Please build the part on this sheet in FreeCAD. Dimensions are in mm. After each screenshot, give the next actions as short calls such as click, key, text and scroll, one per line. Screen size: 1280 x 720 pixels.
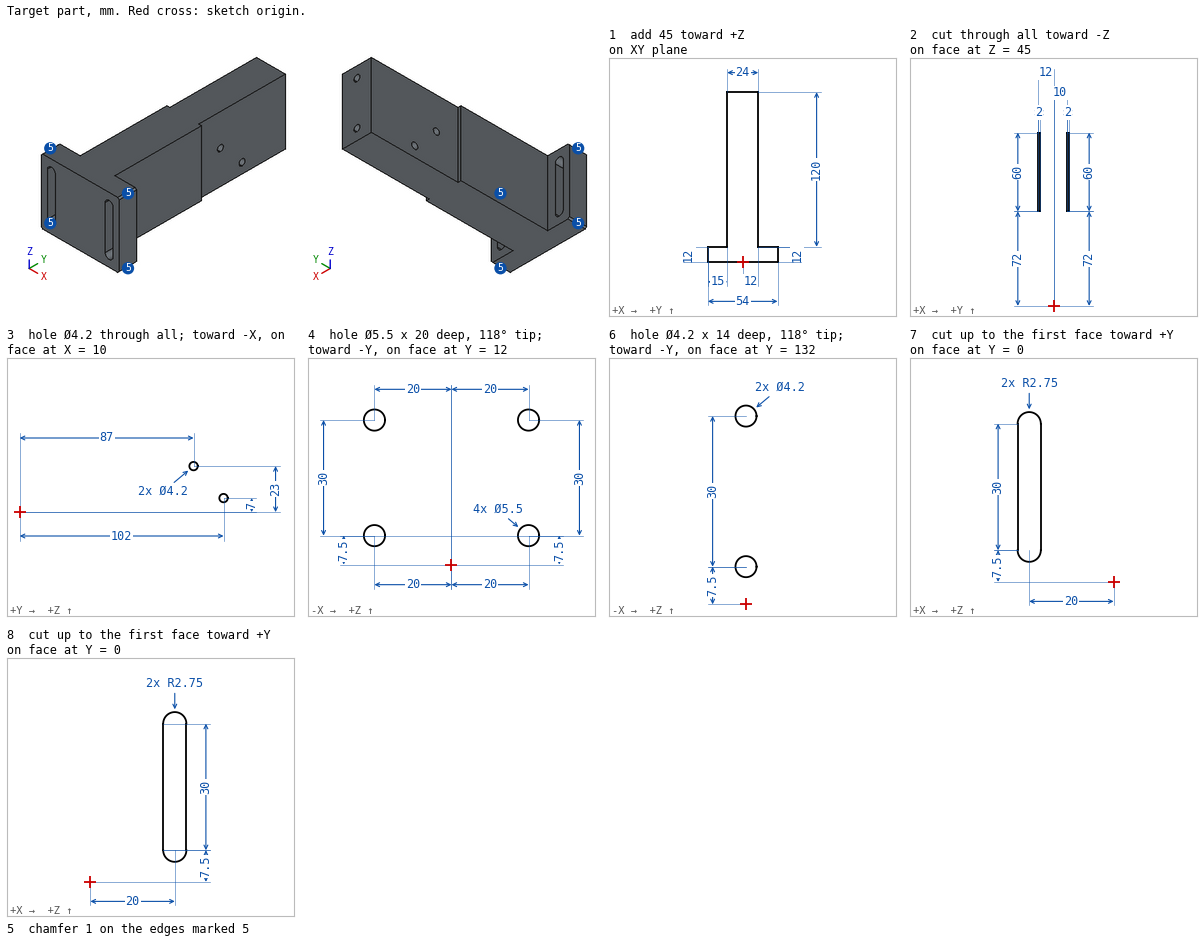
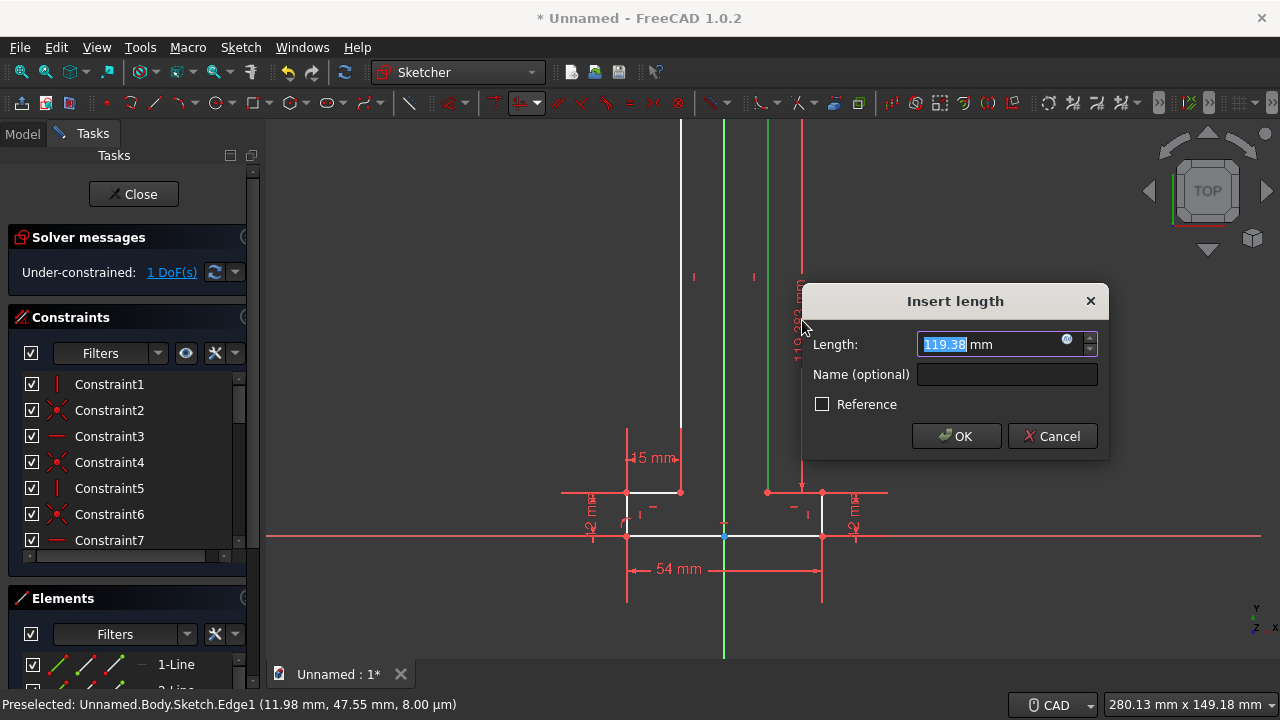
text(120)
key(Return)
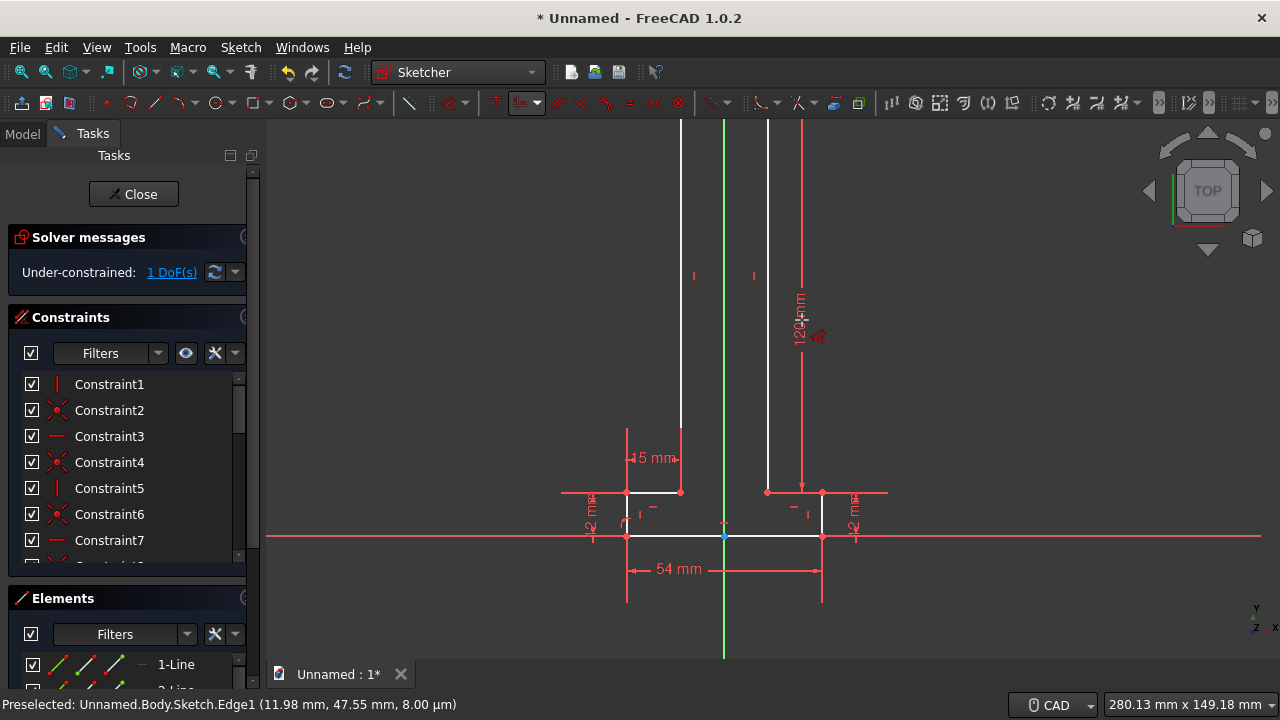
click(768, 493)
click(756, 570)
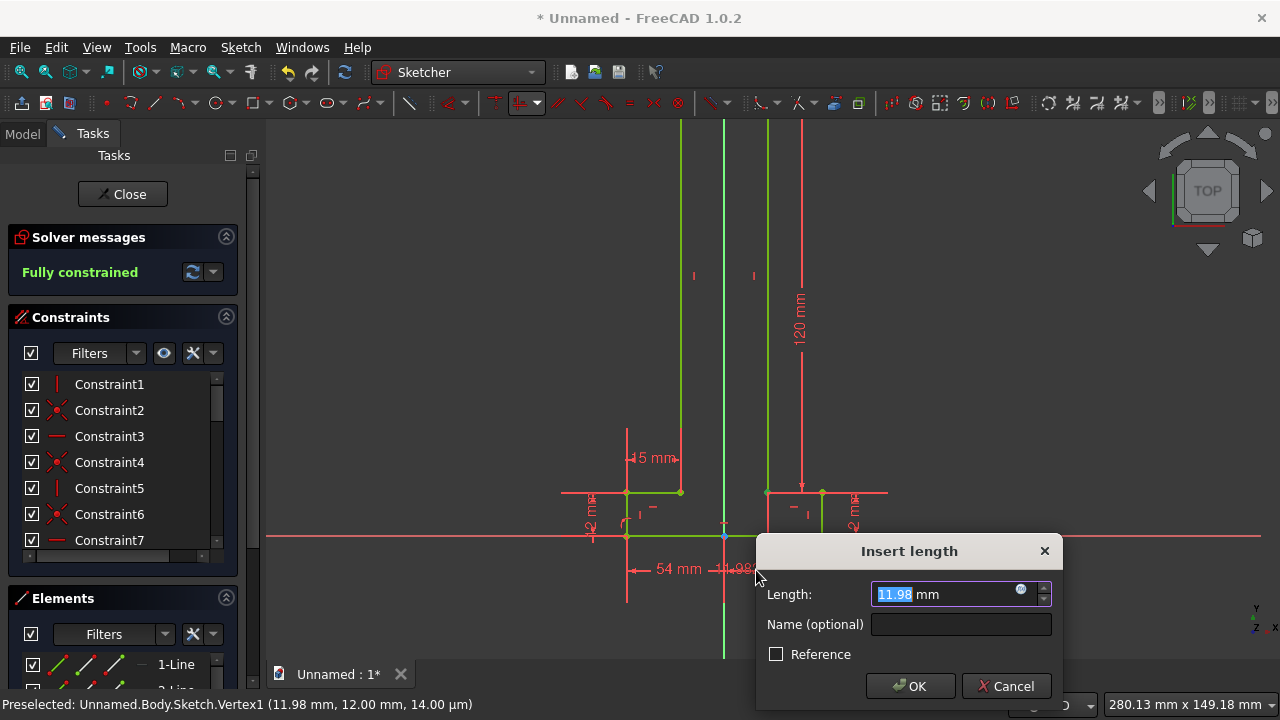
text(12)
key(Return)
key(Escape)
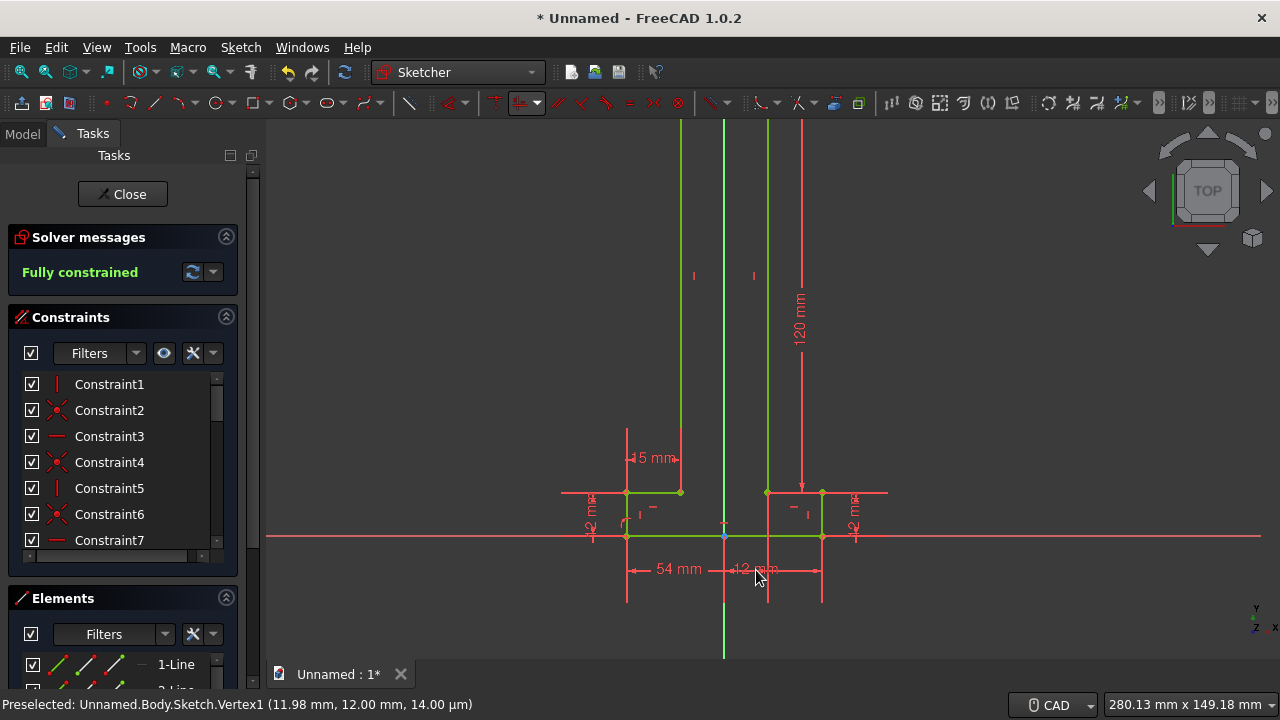
click(123, 194)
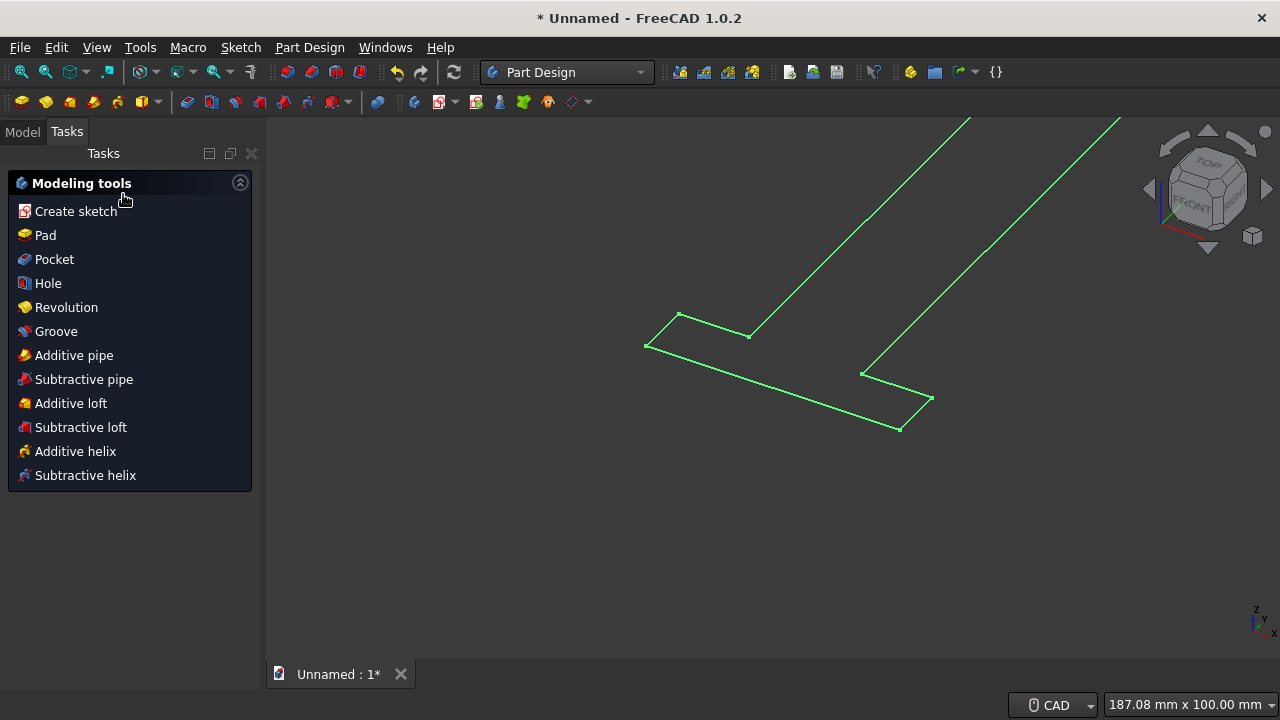
click(22, 102)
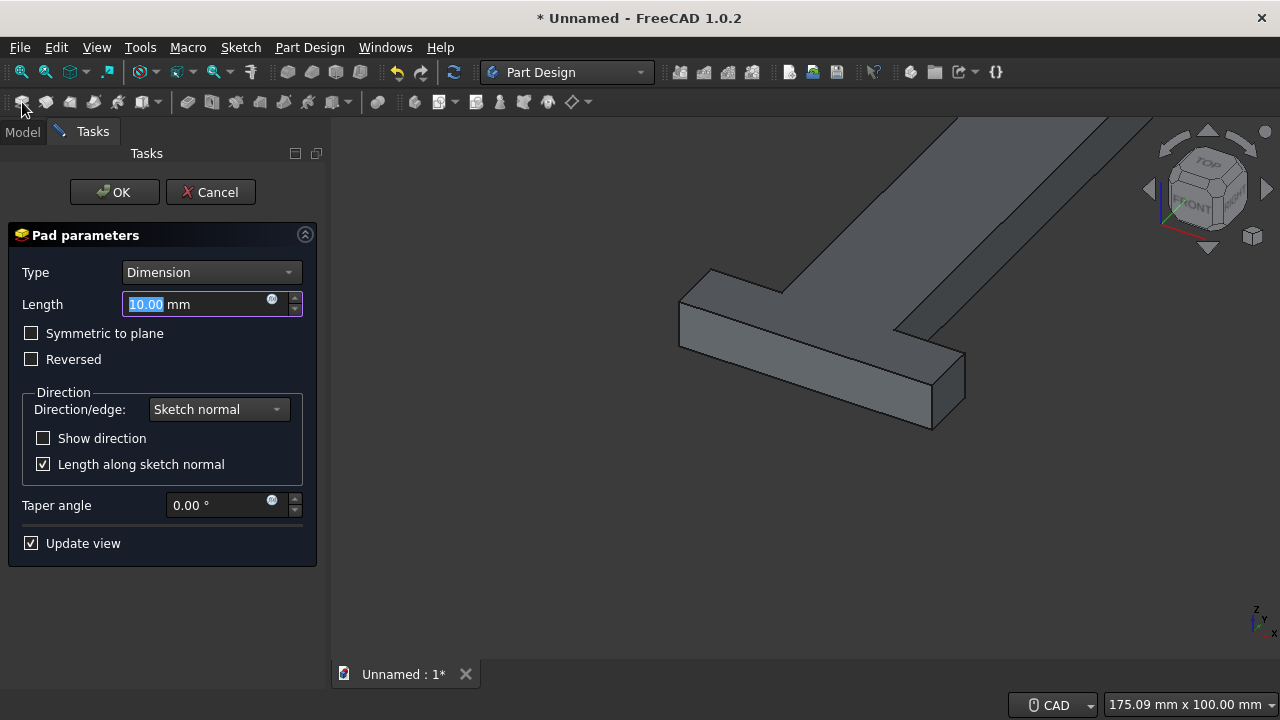
text(45)
key(Tab)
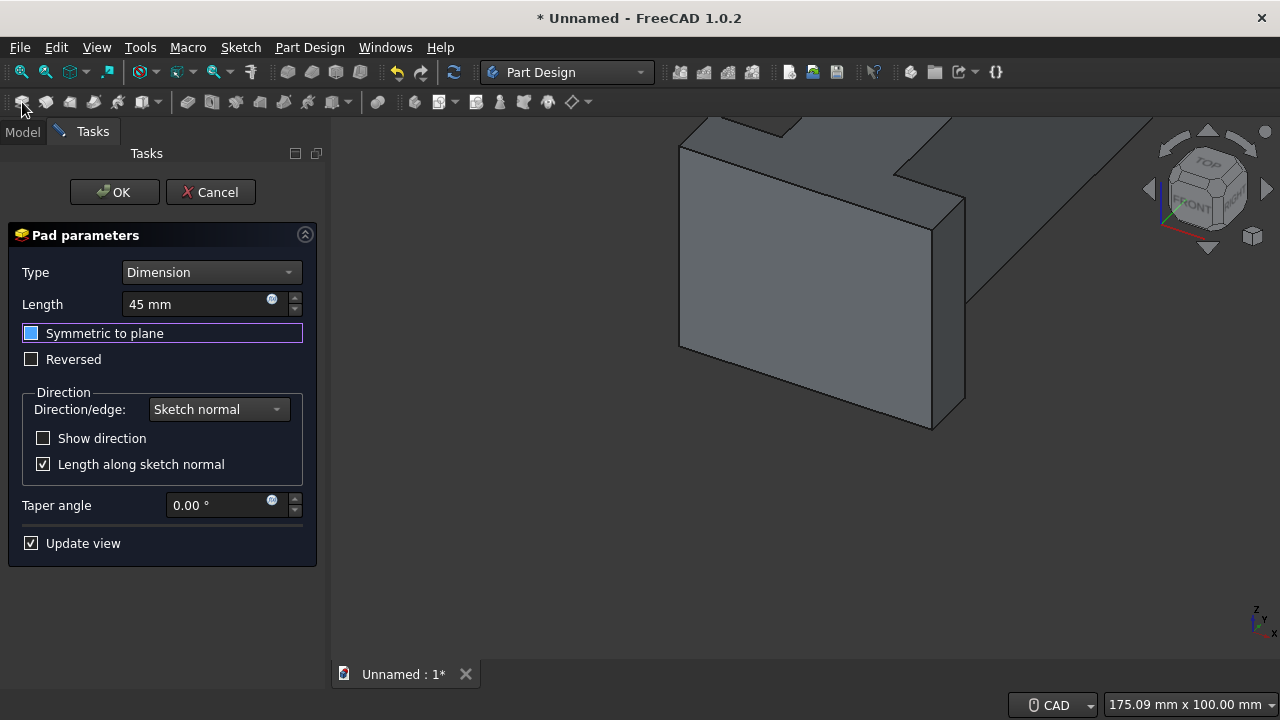
click(115, 192)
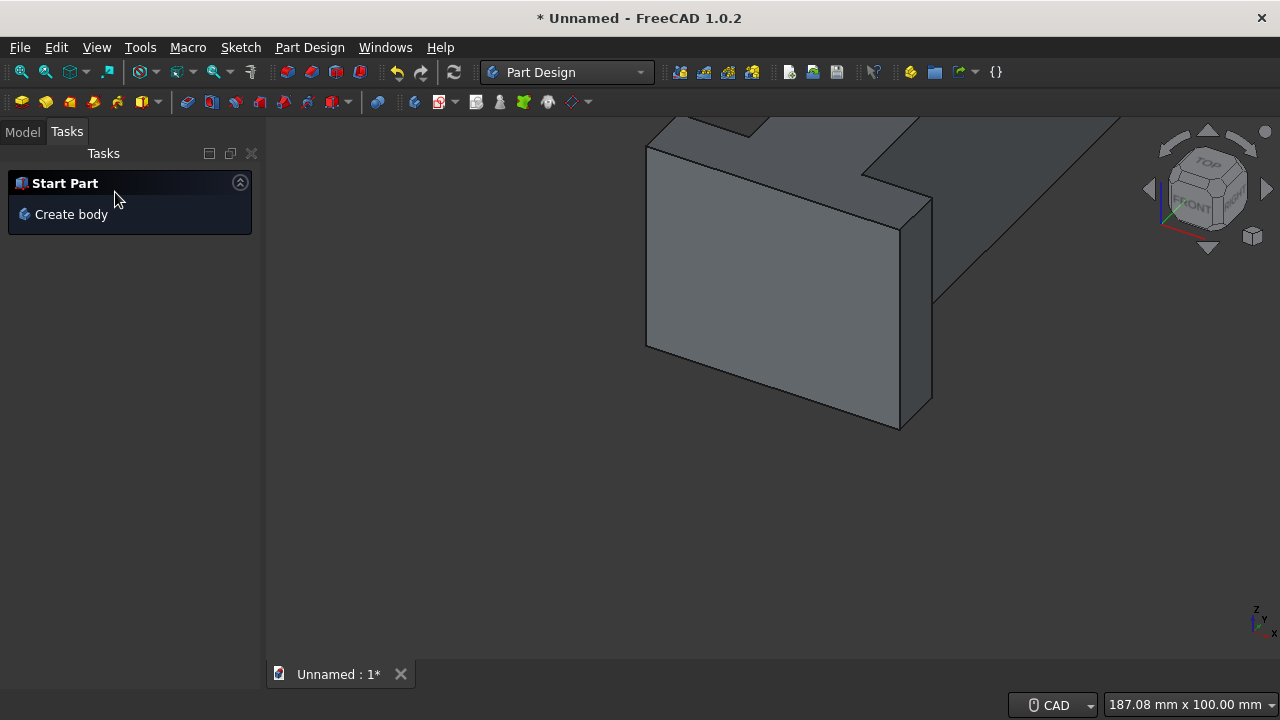
click(22, 72)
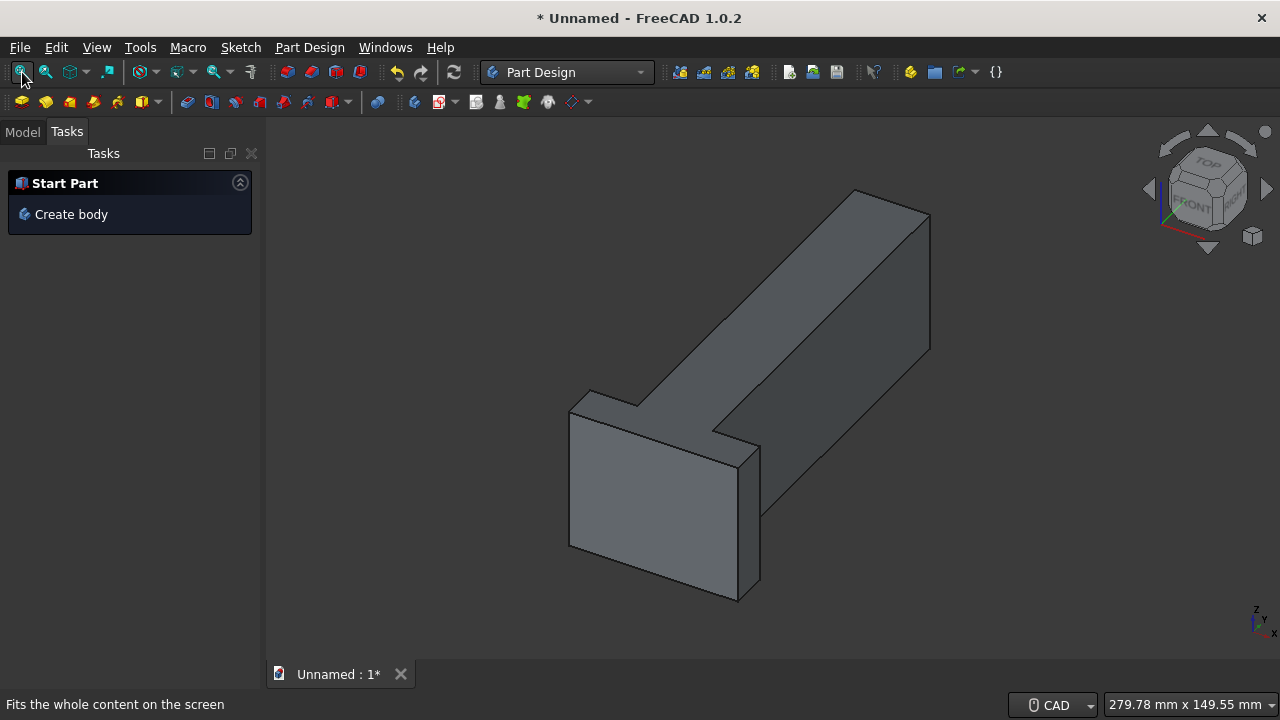
click(841, 252)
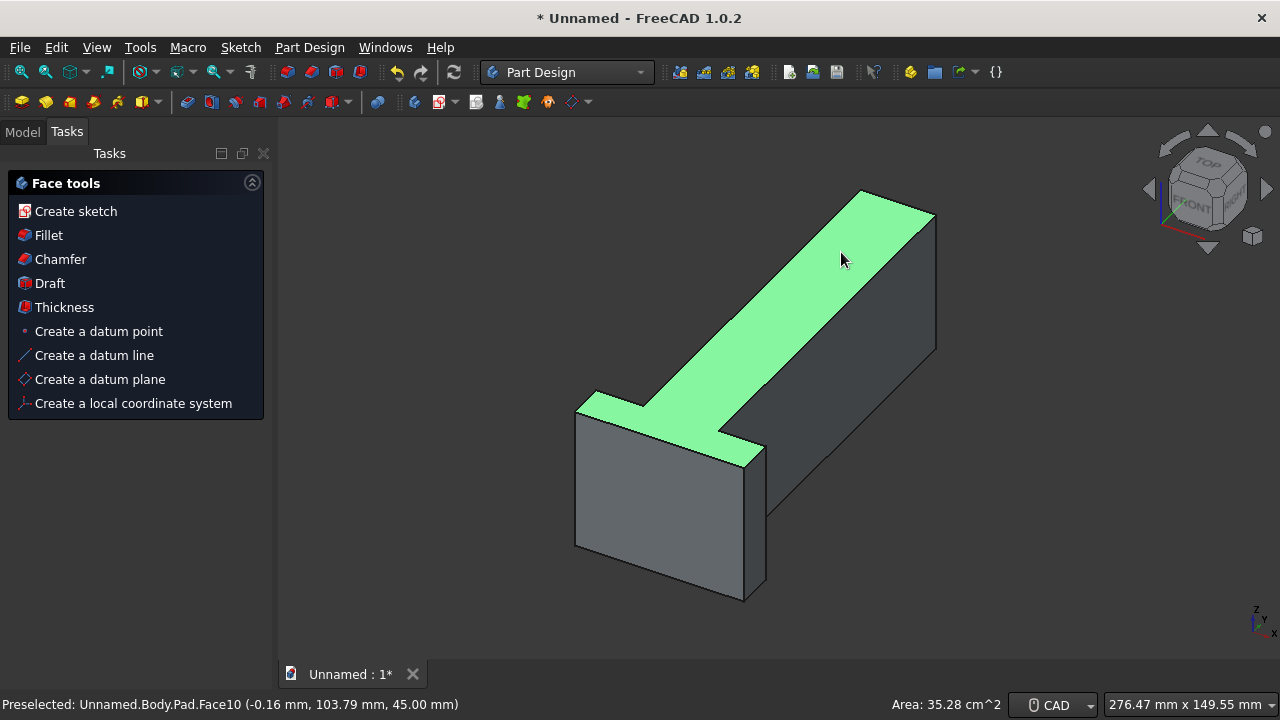
click(440, 102)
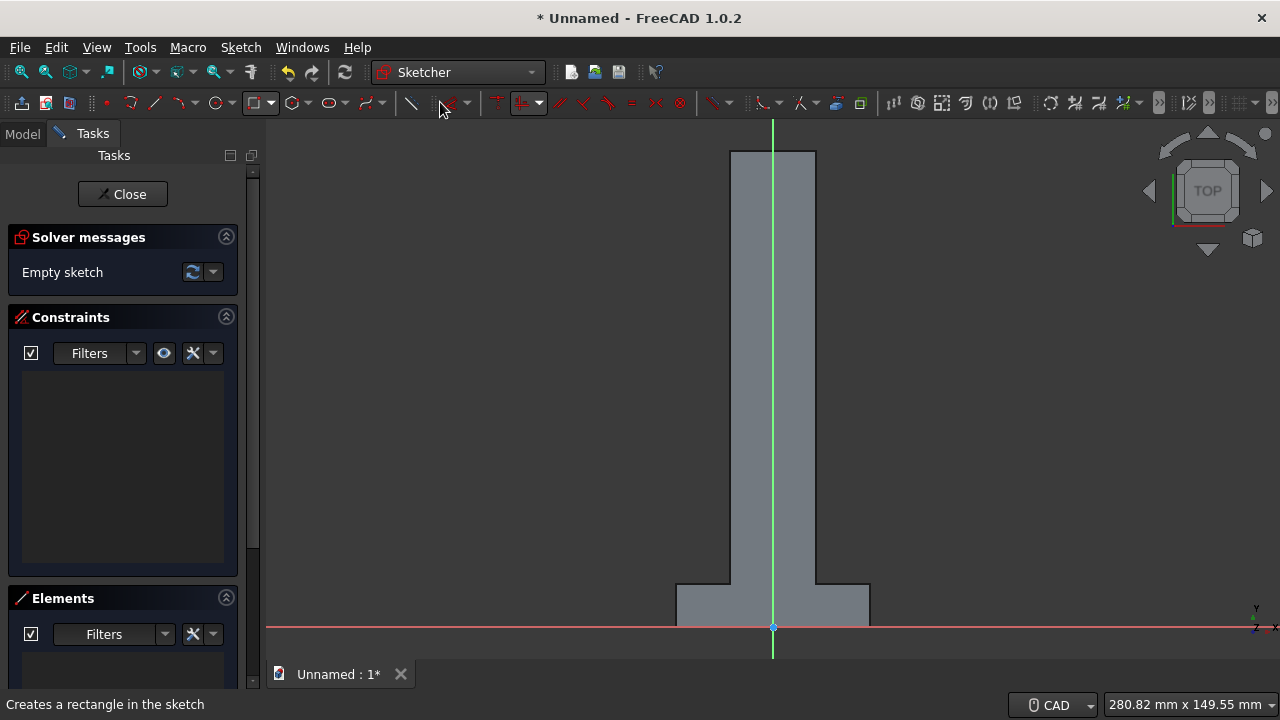
scroll(565, 389, down, 2)